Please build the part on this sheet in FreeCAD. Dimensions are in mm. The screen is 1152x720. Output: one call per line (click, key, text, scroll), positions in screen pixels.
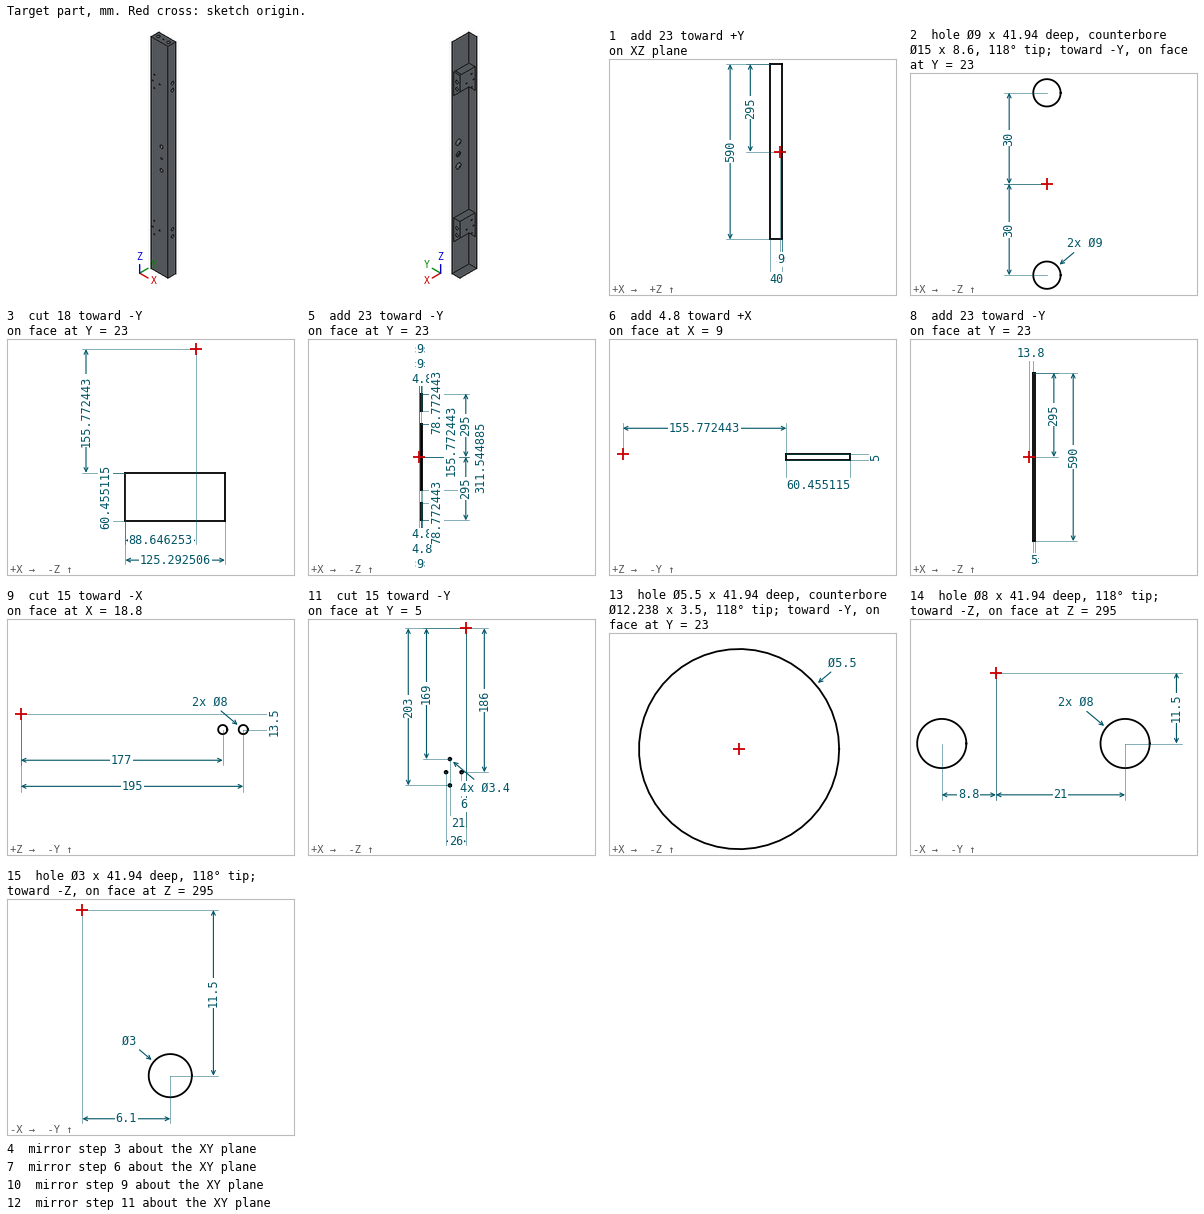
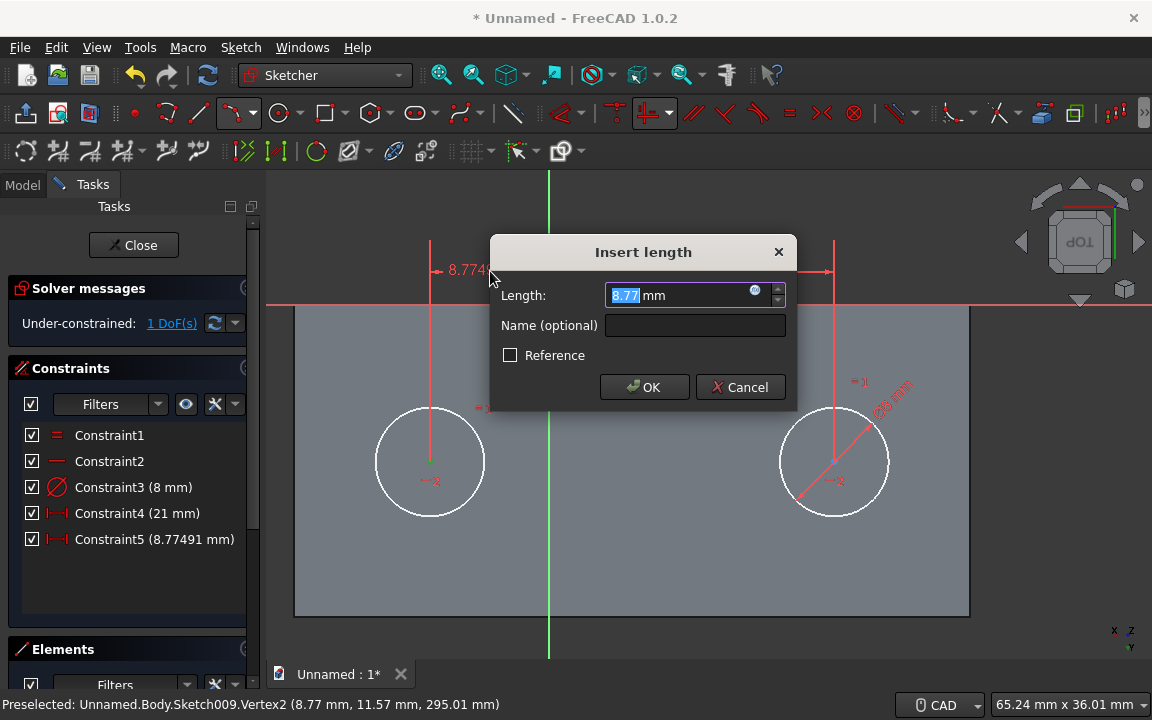
text(8.8)
key(Return)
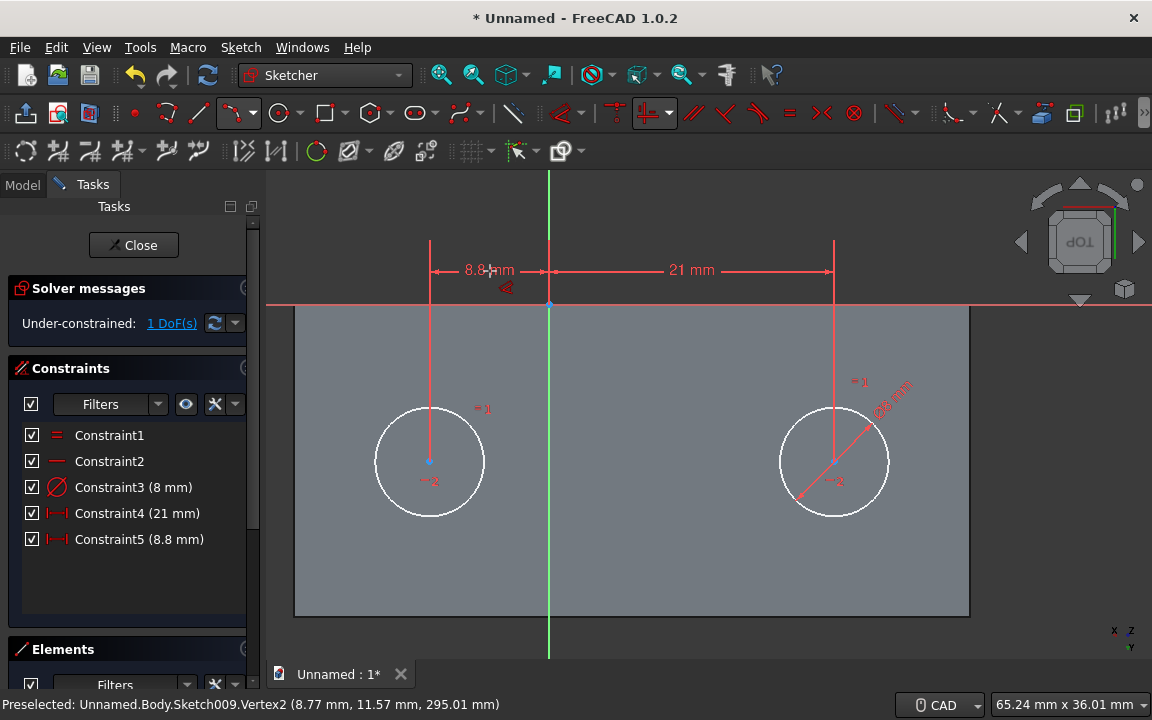
click(834, 462)
click(868, 347)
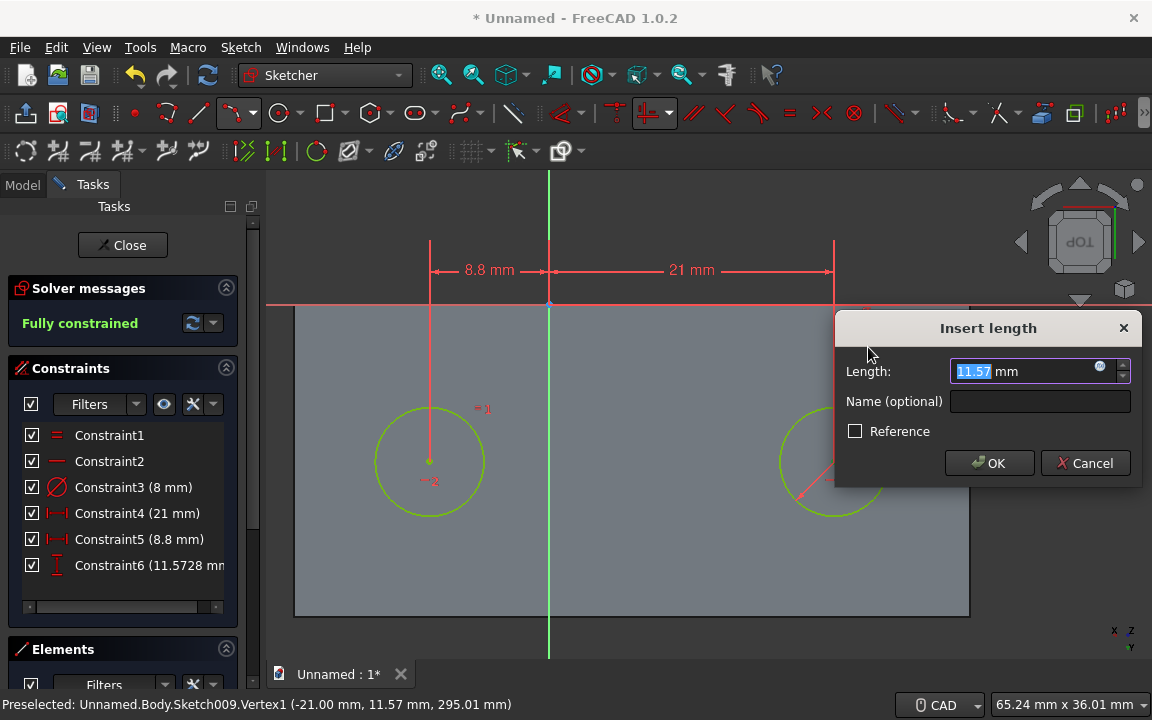
text(11.5)
key(Return)
key(Escape)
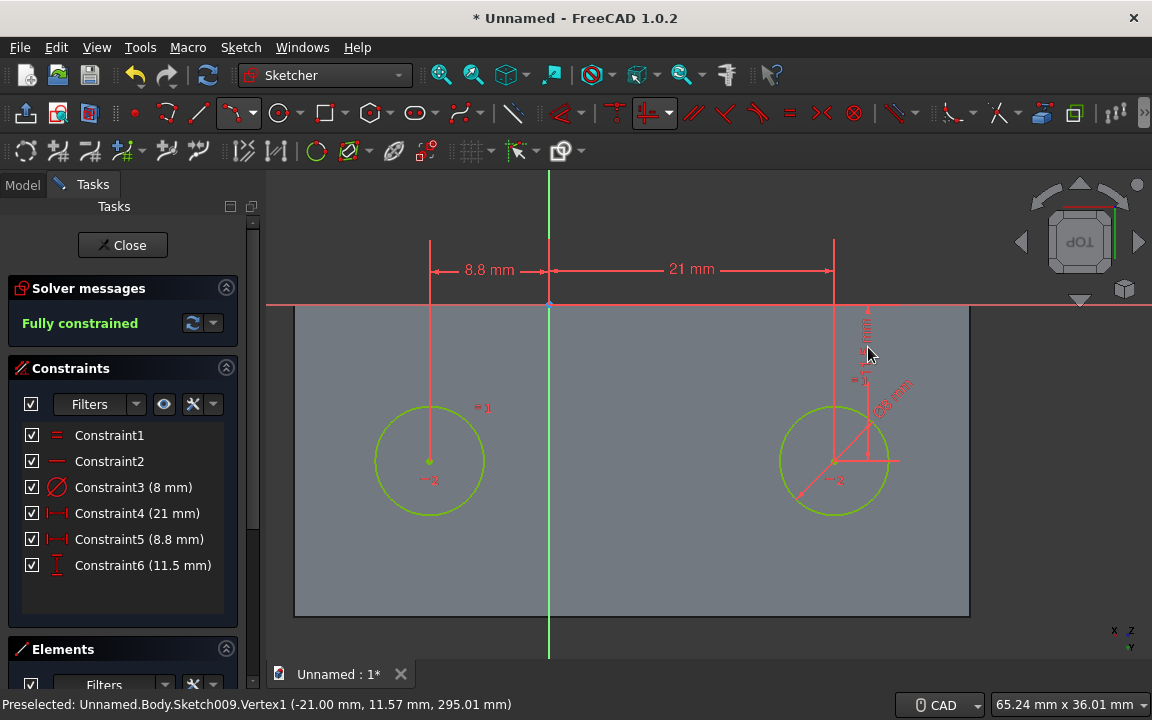
click(123, 245)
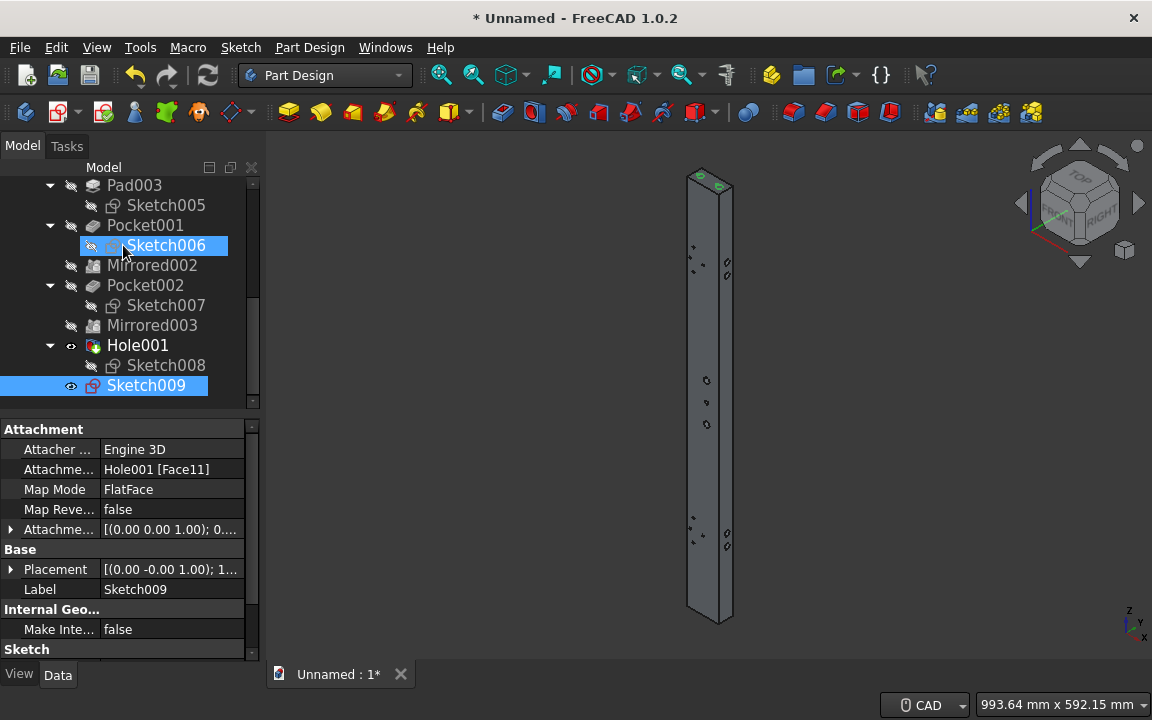
click(536, 112)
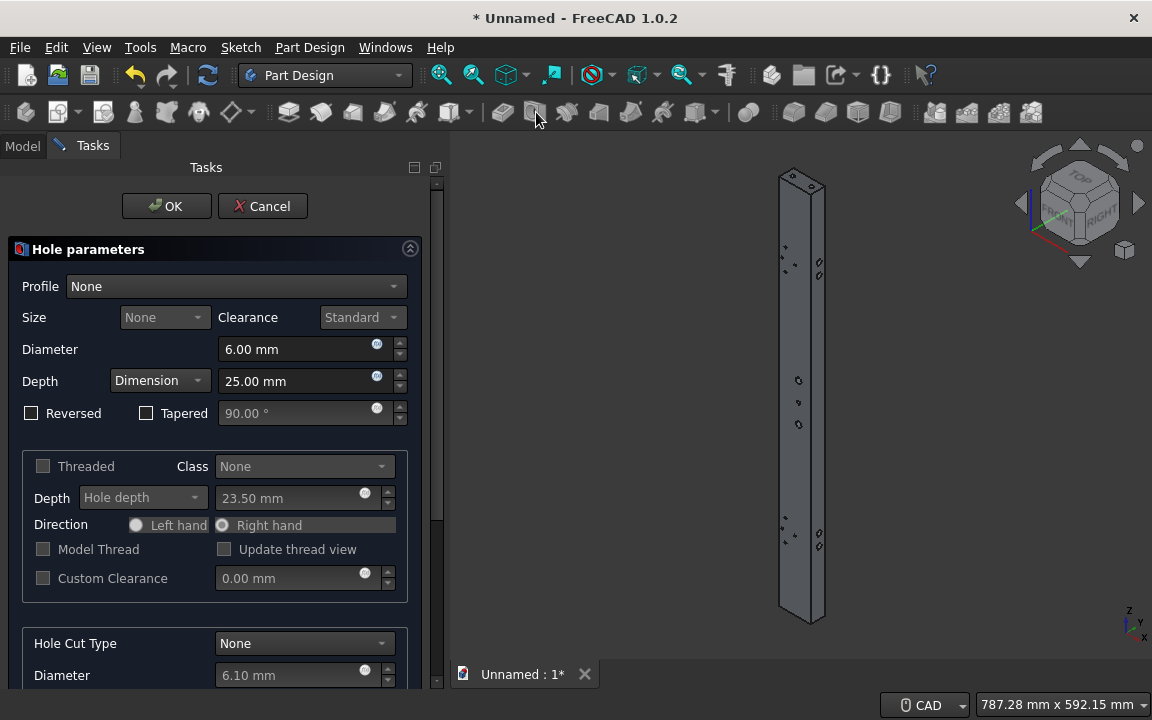
triple_click(305, 349)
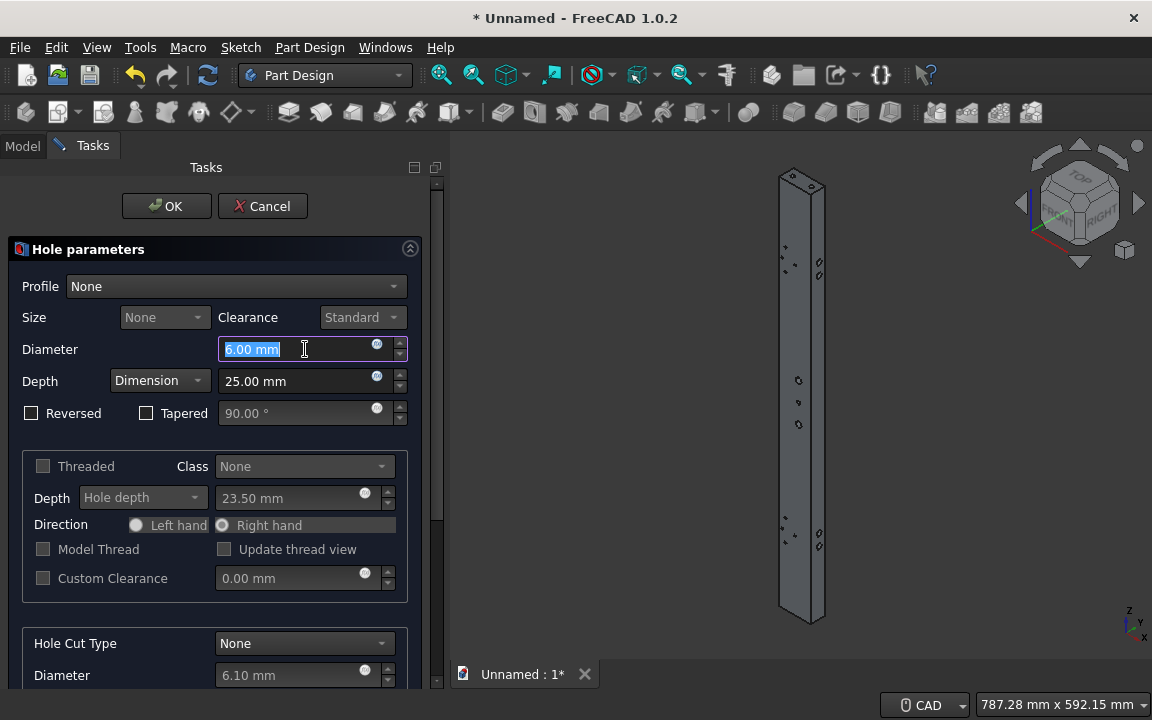
text(8)
key(Tab)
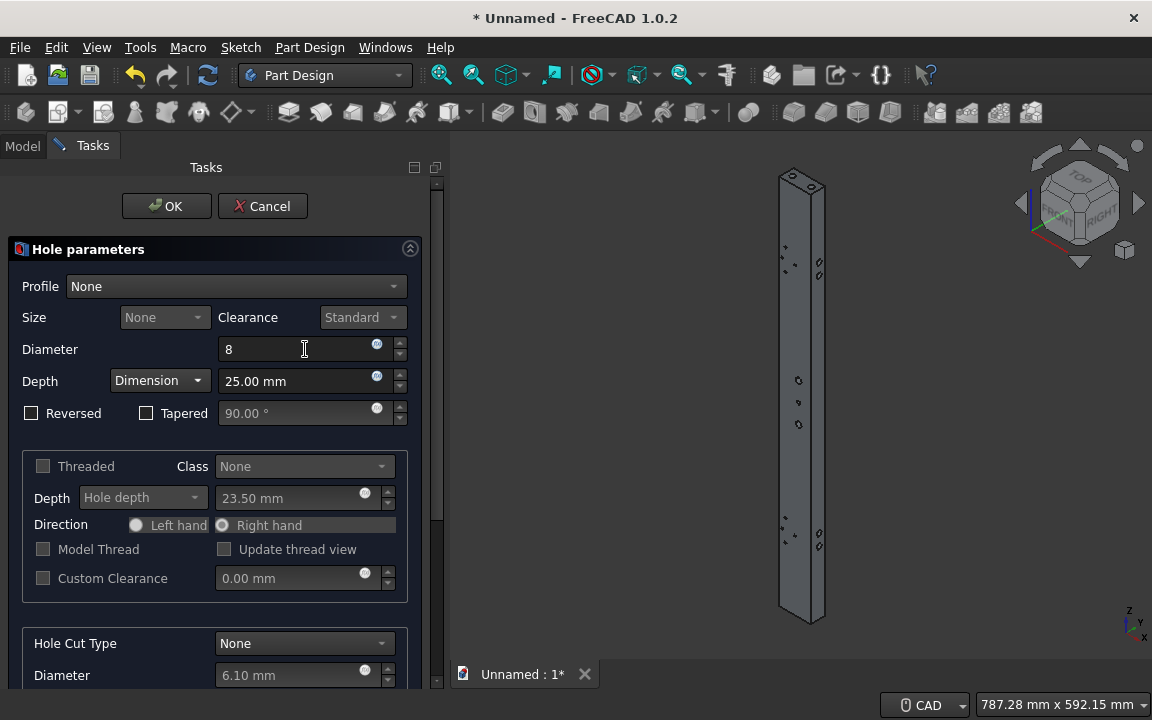
triple_click(305, 381)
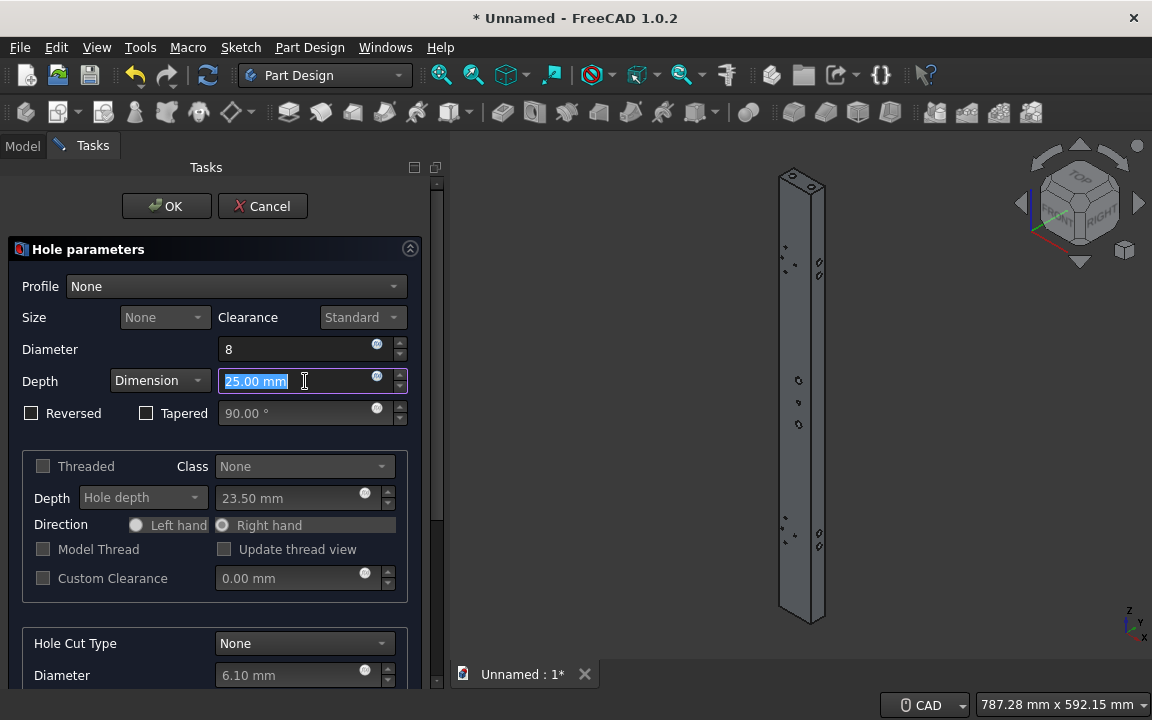
text(41.94)
key(Tab)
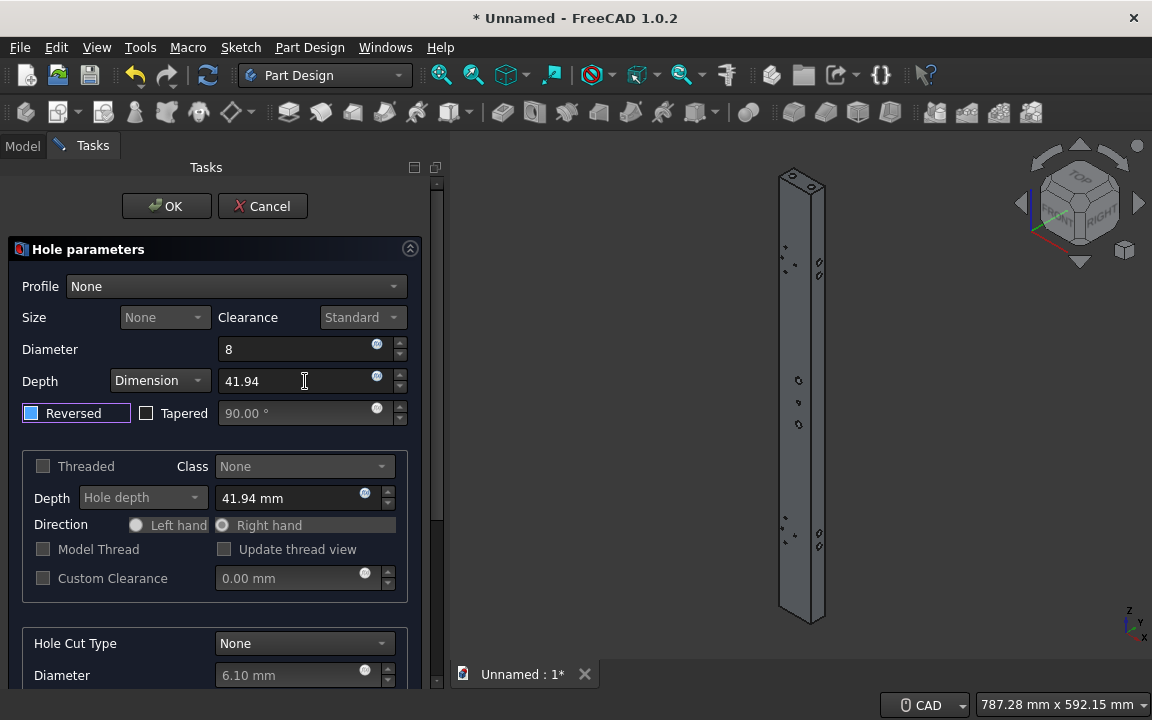
click(167, 206)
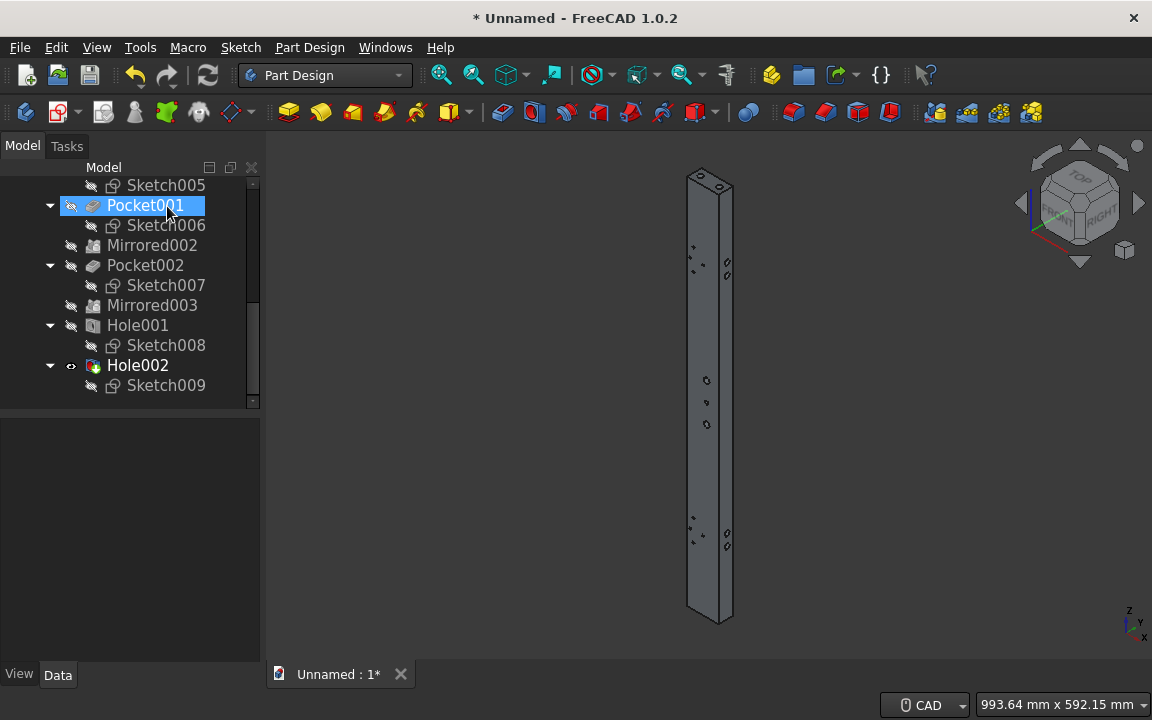
key(2)